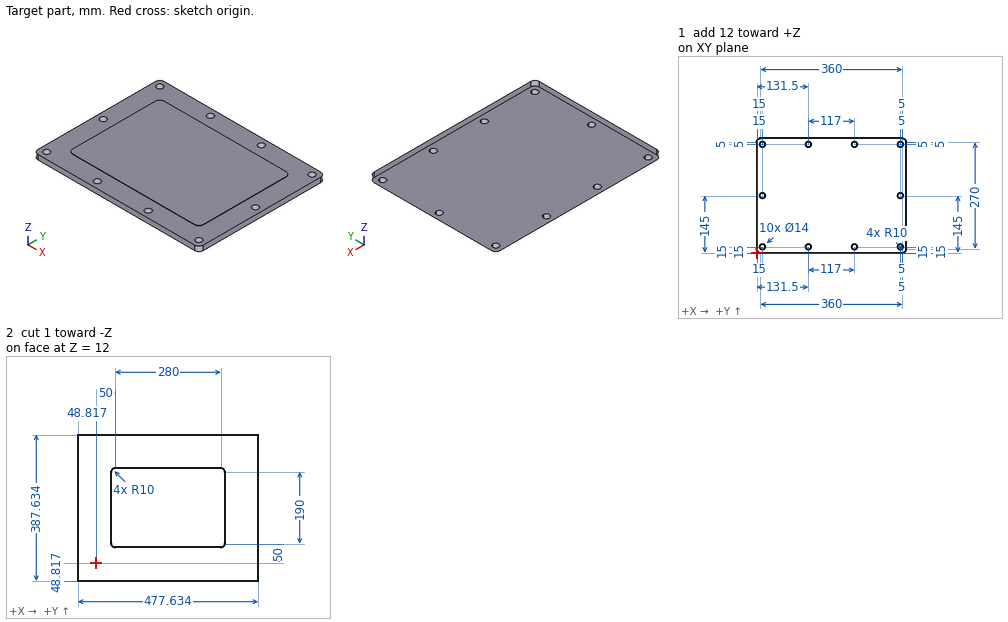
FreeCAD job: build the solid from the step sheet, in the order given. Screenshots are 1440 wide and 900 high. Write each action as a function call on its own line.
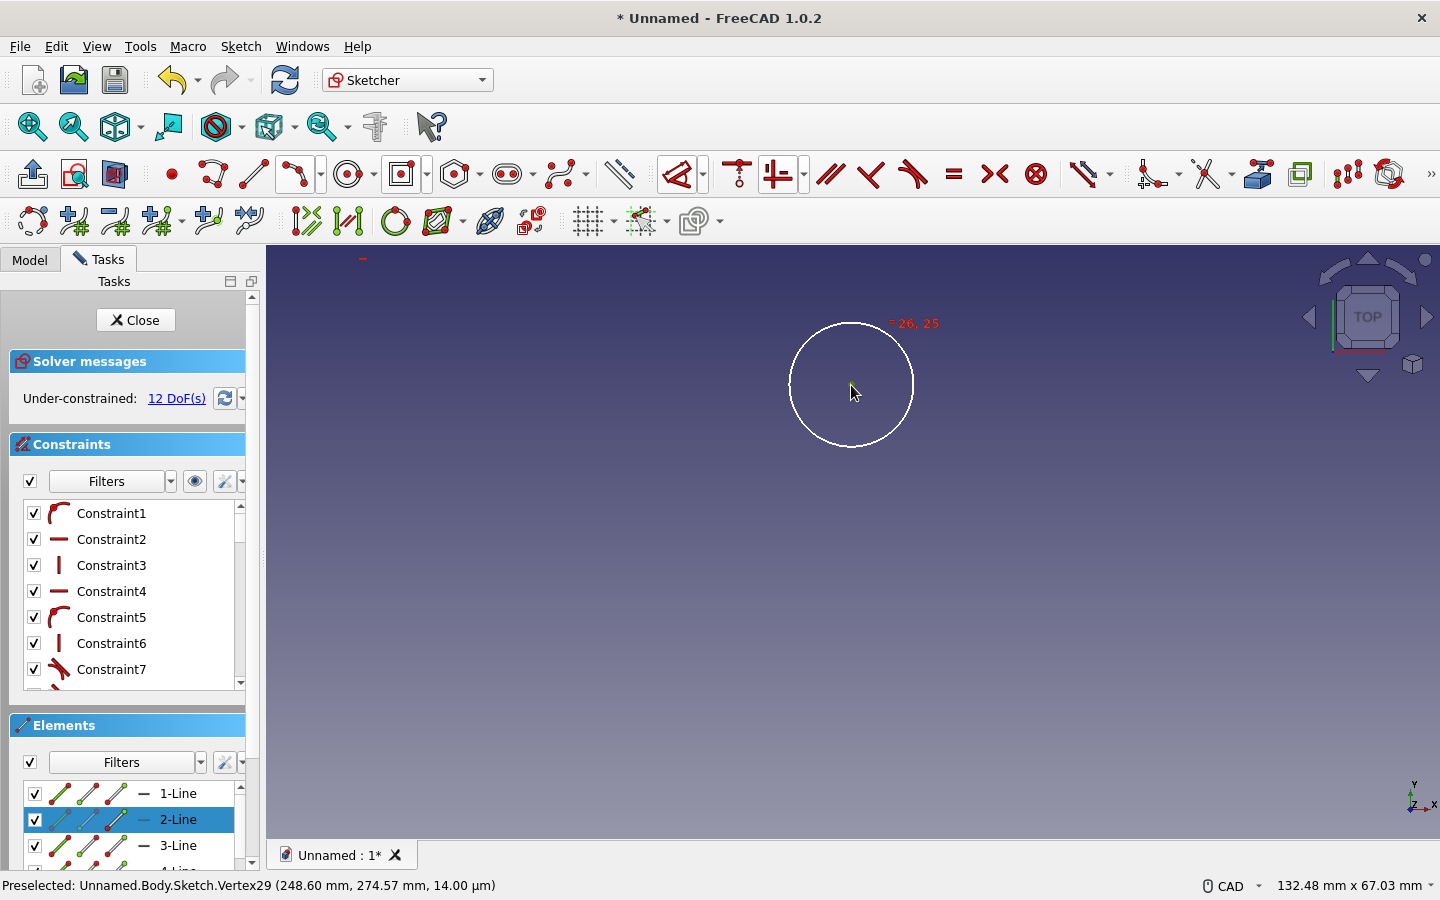
click(702, 174)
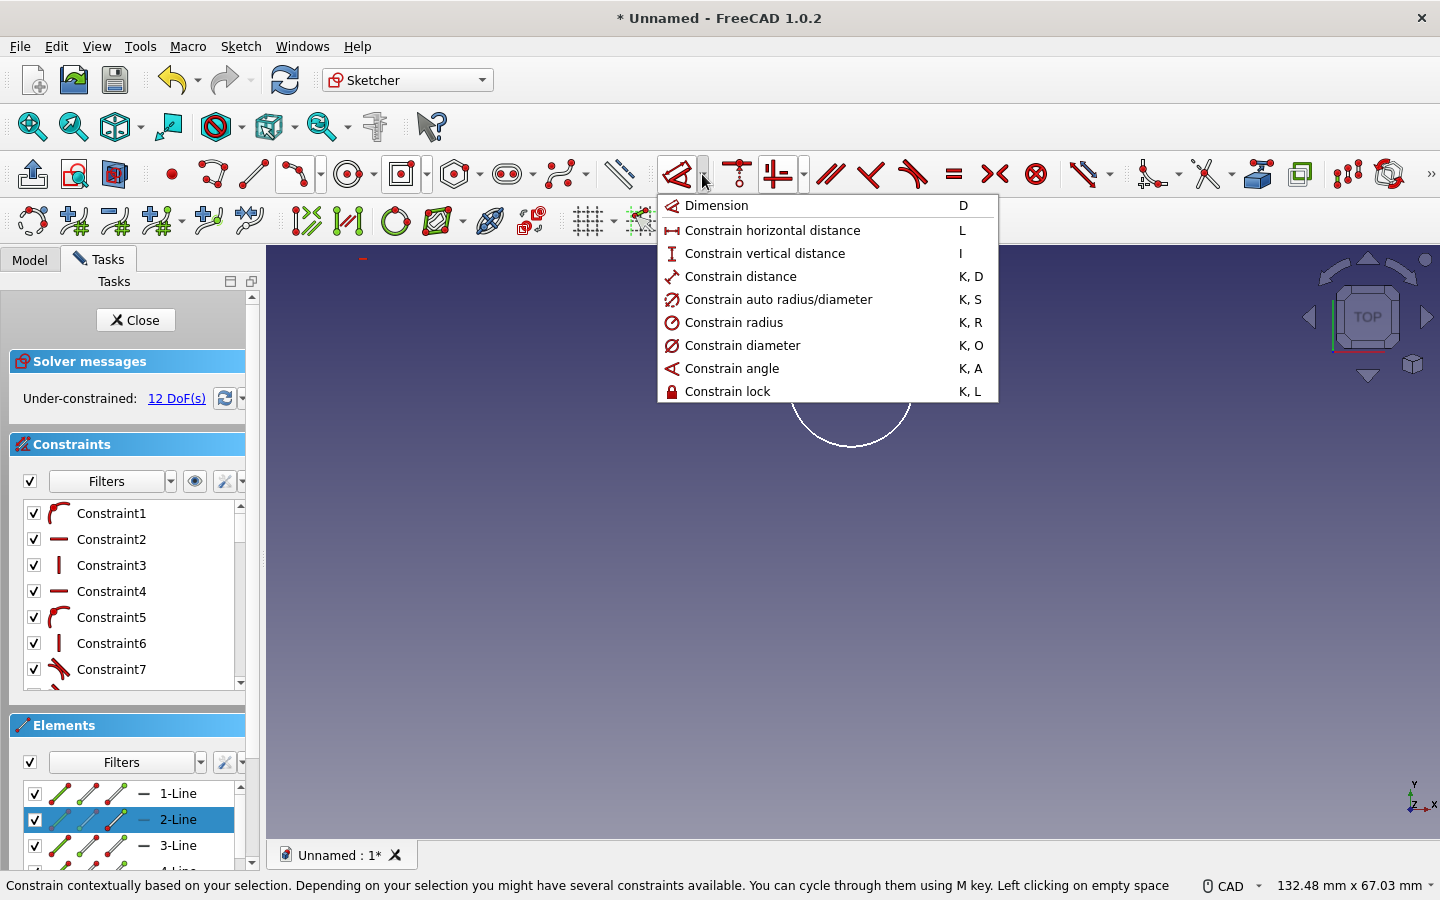
click(828, 254)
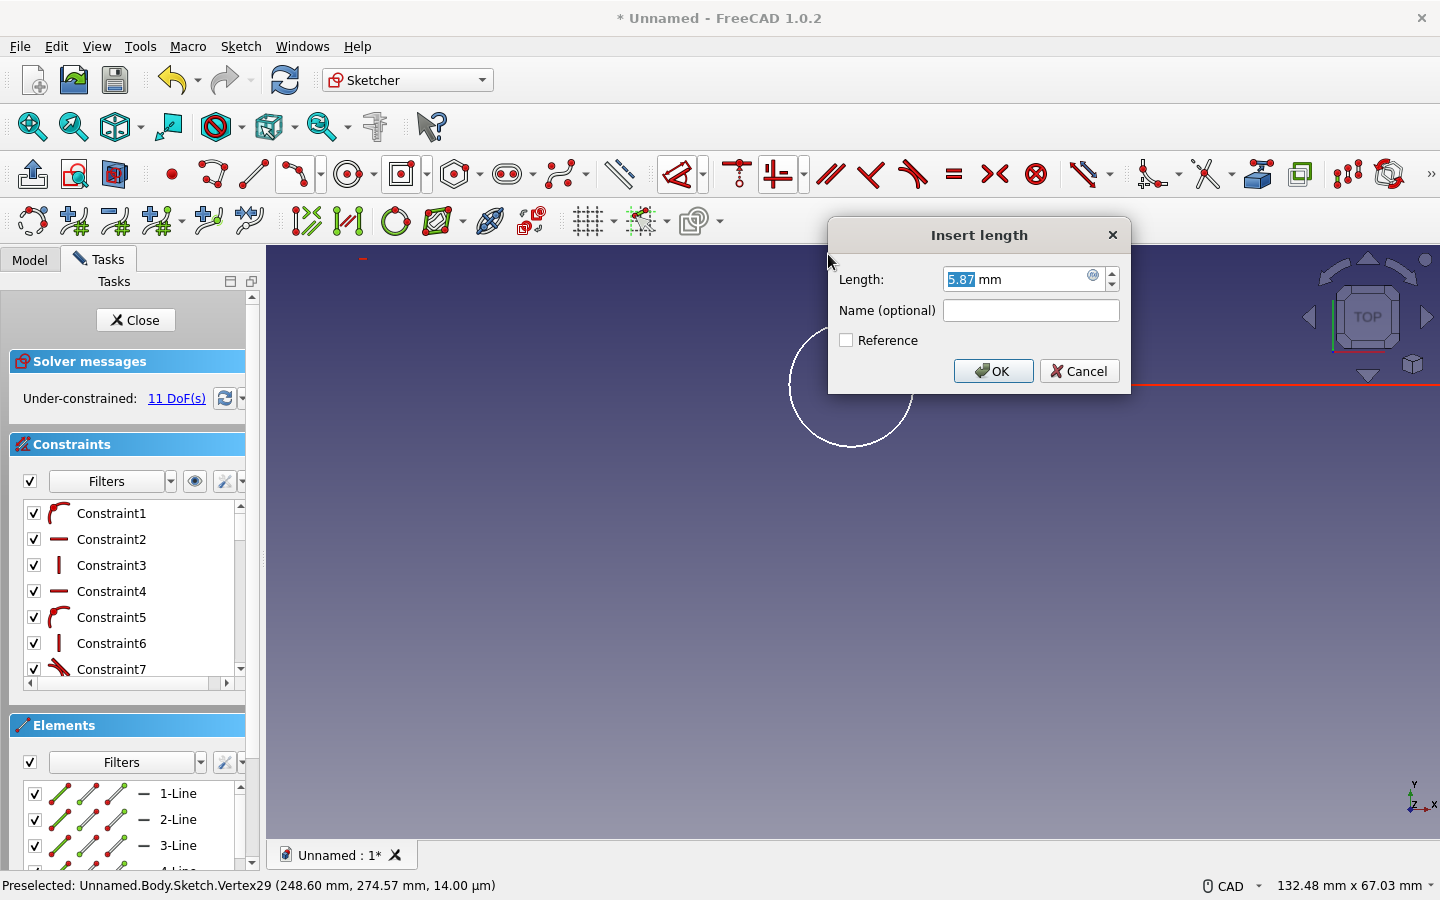
text(5)
key(Return)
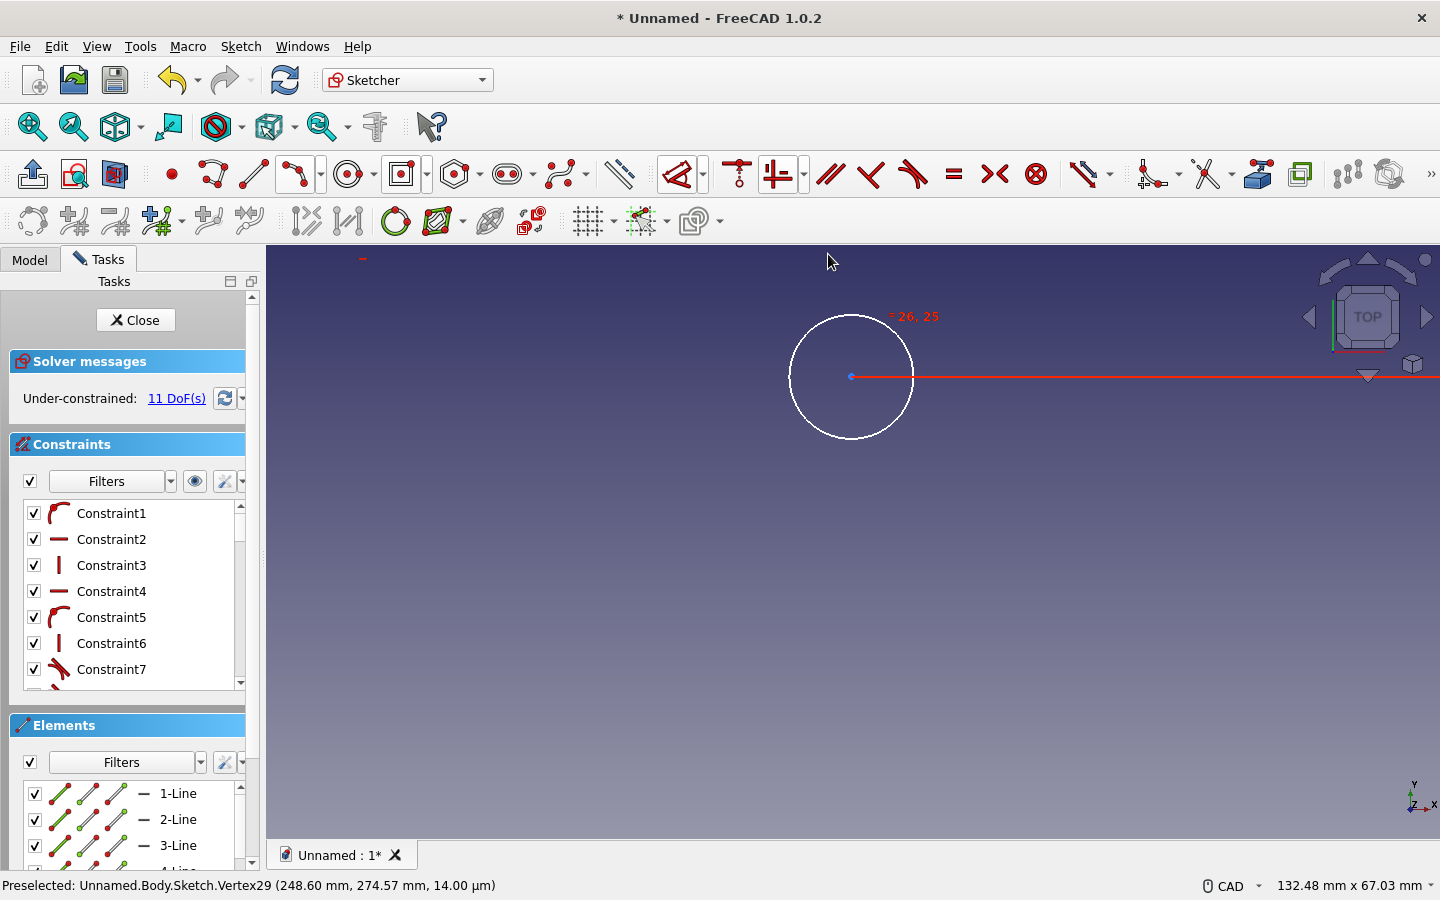
scroll(855, 387, down, 10)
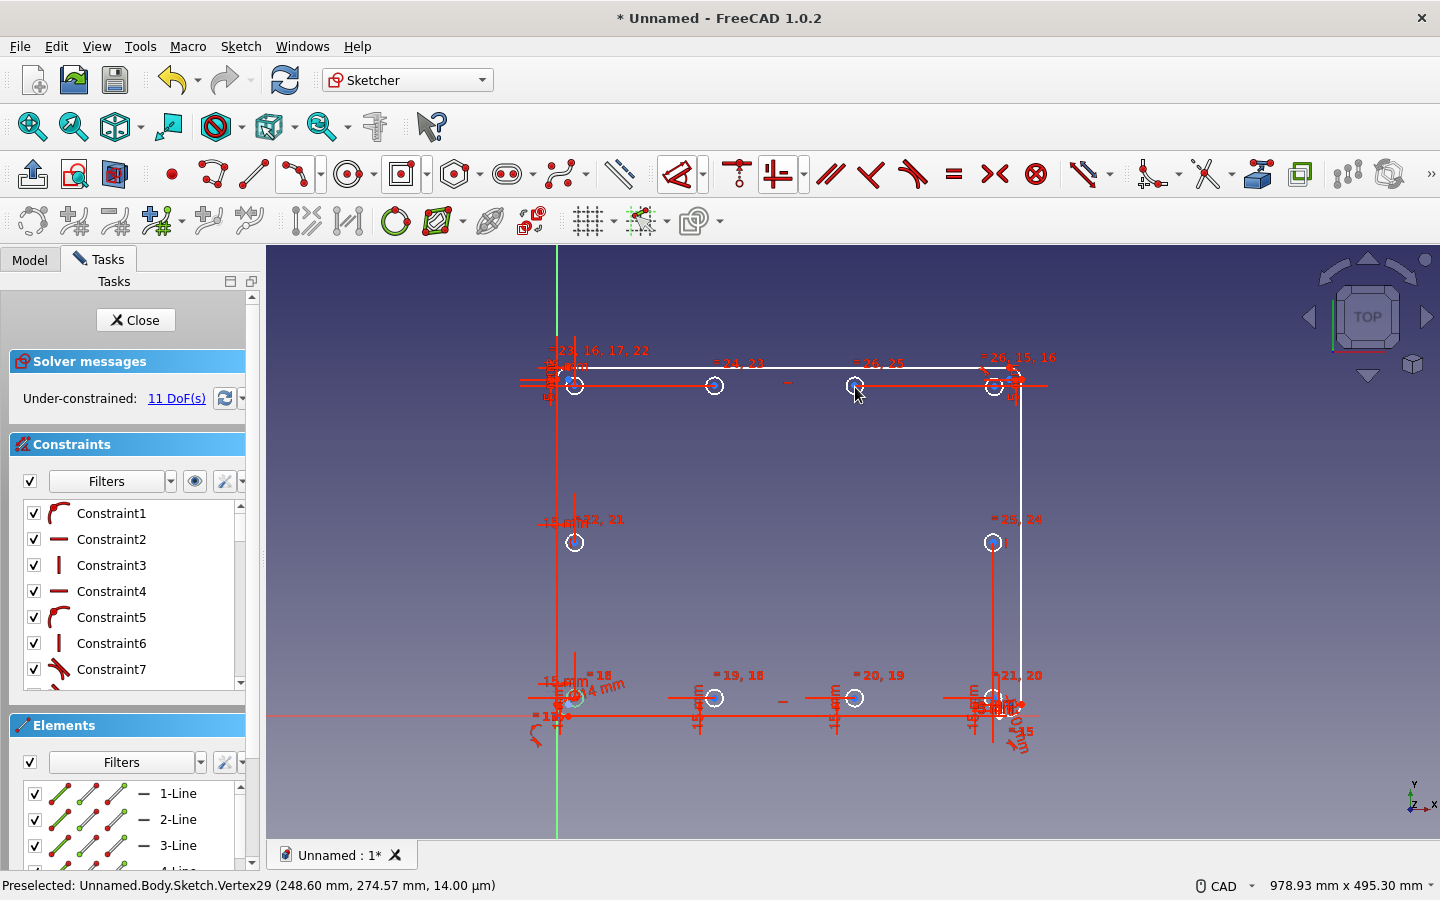
scroll(1009, 368, up, 10)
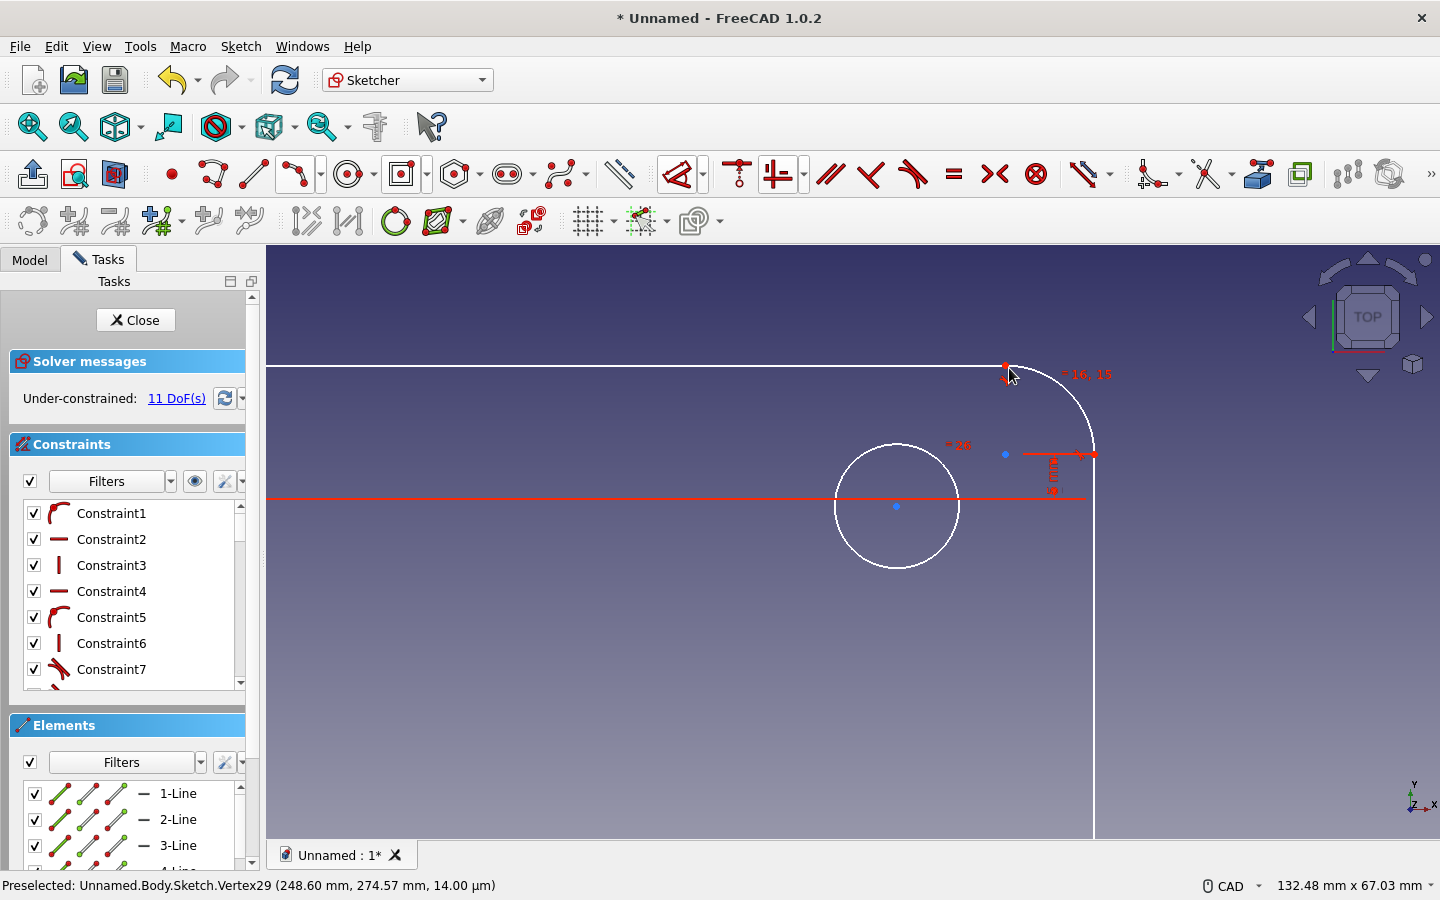
click(1006, 366)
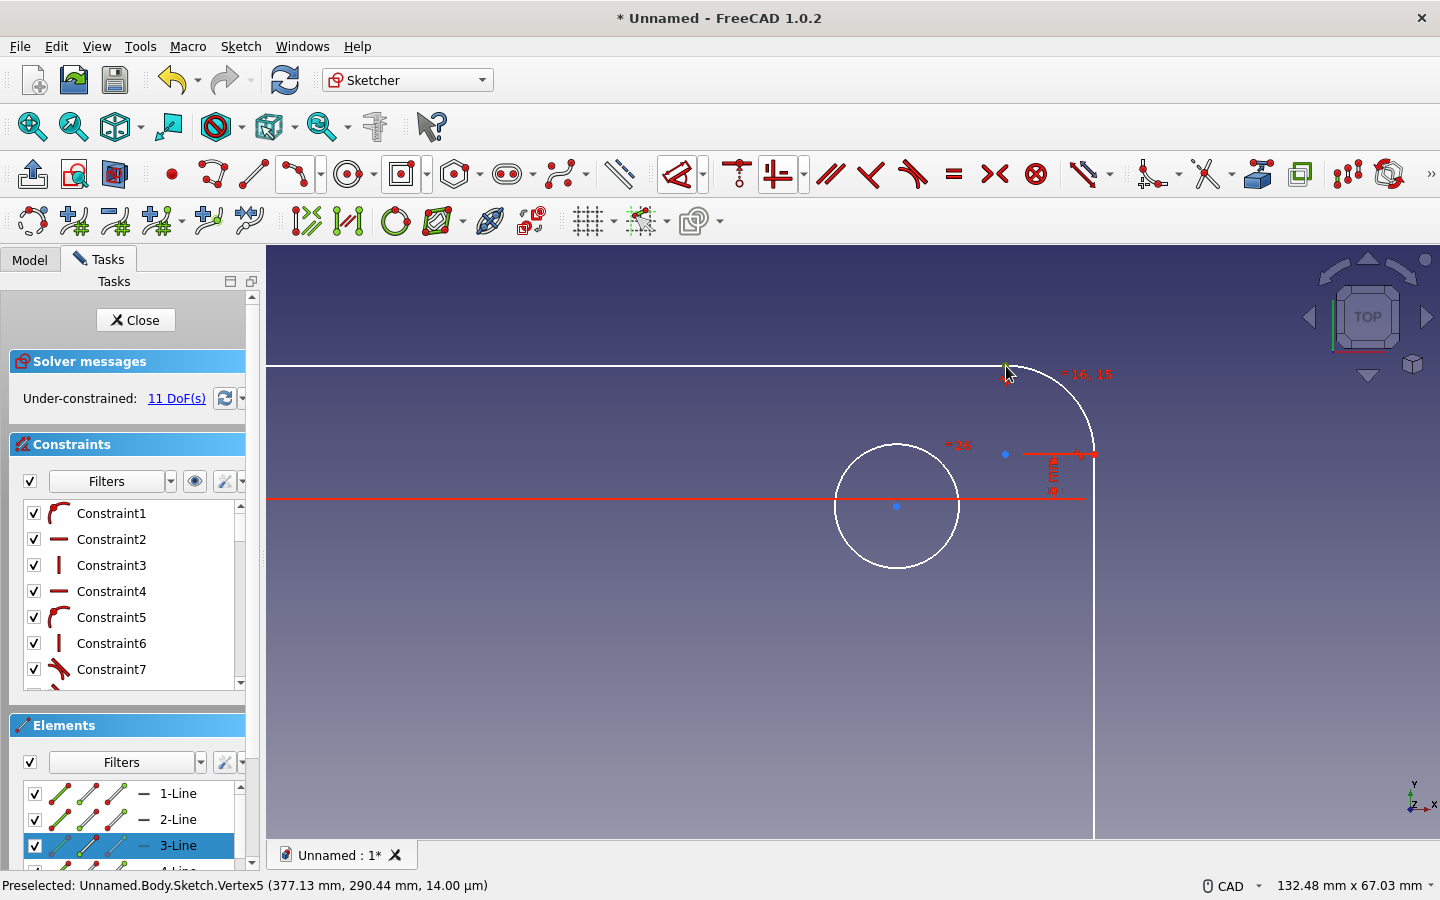
click(897, 506)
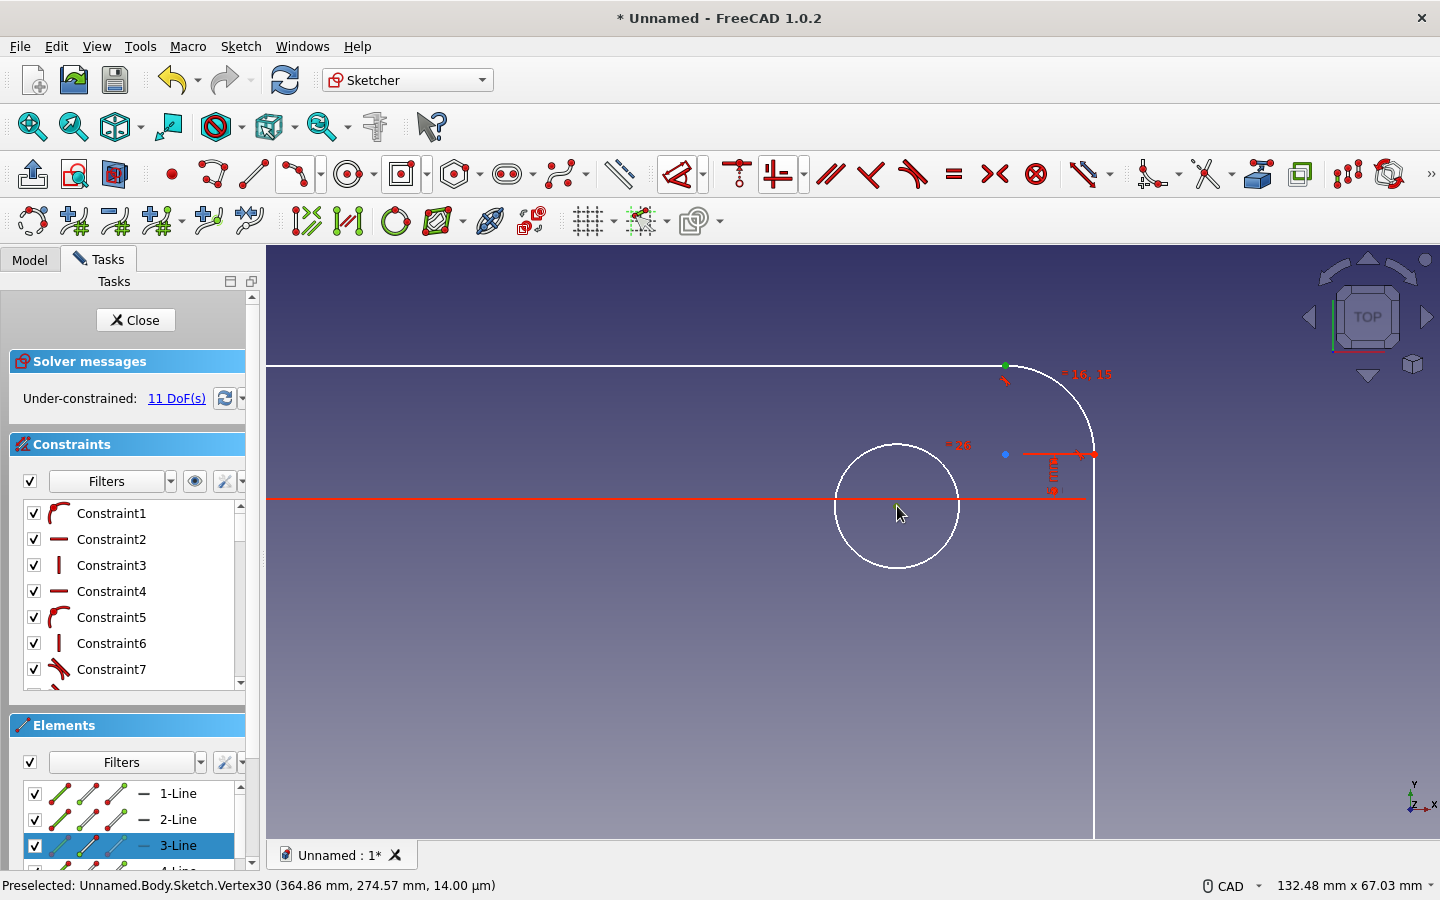
key(l)